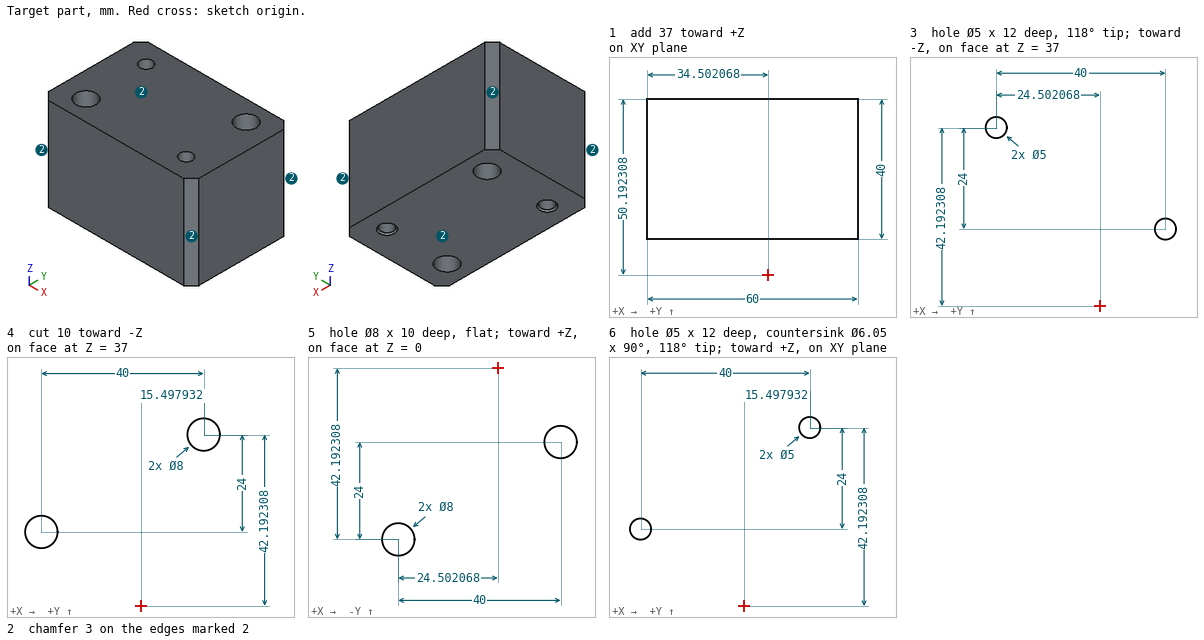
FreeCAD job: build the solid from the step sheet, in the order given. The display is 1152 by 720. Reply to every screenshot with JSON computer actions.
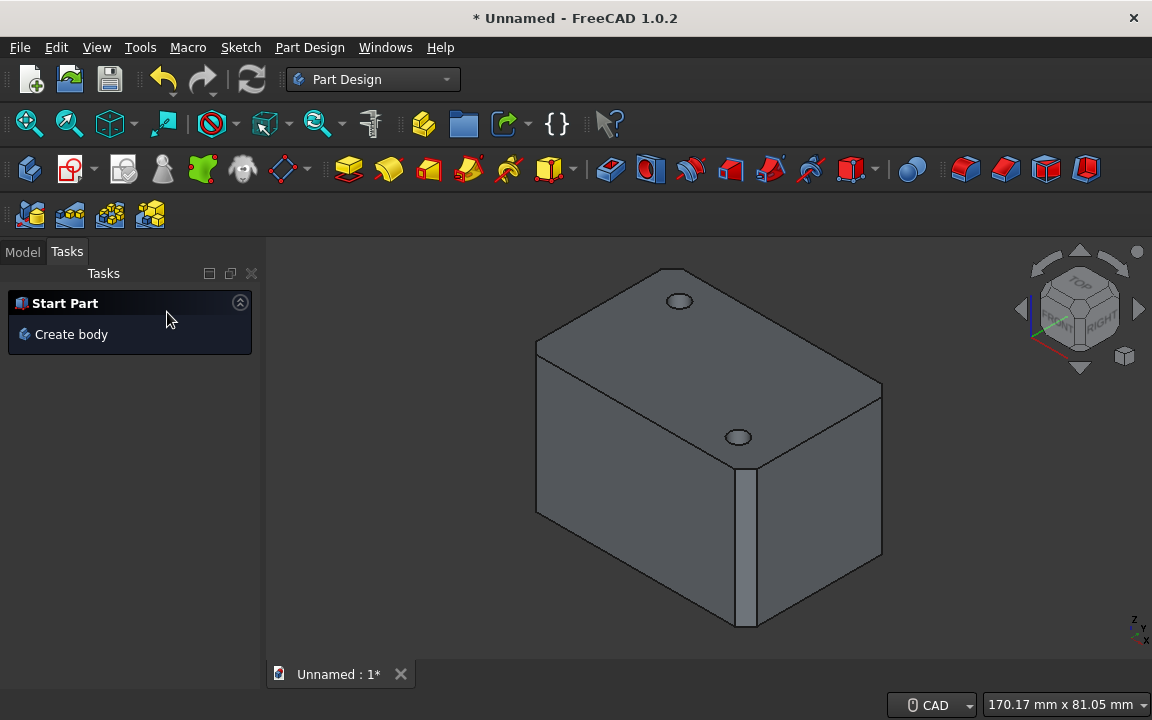
{"action": "left_click", "coordinate": [709, 368]}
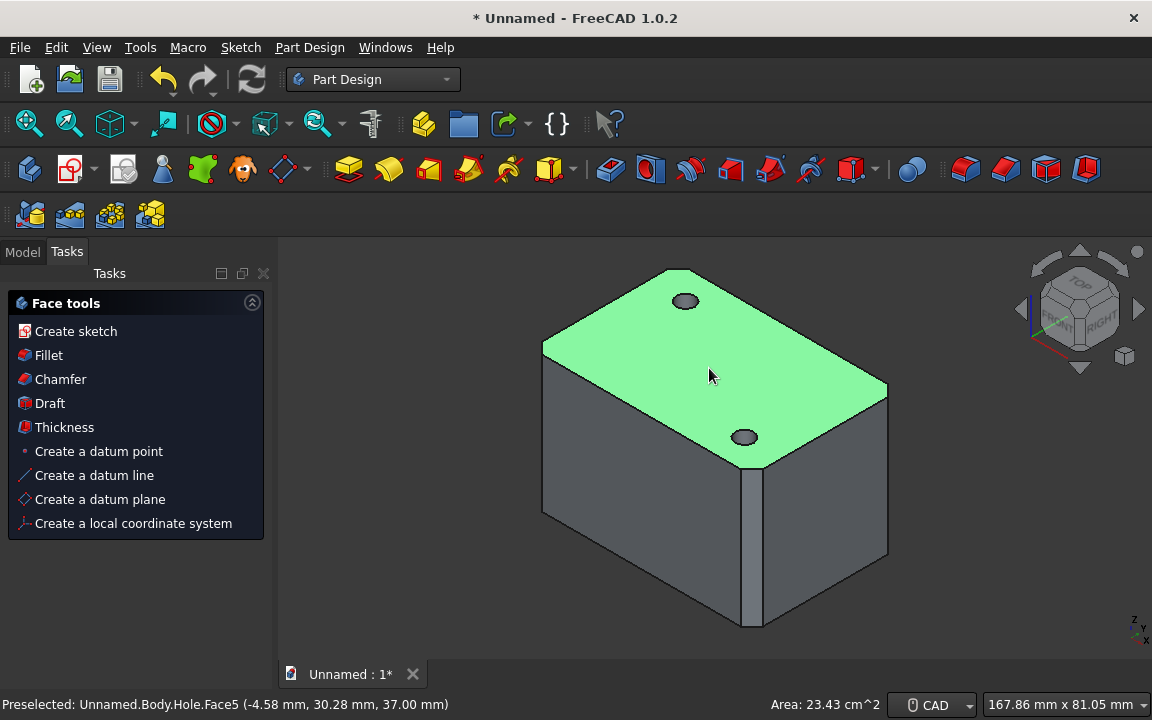
{"action": "left_click", "coordinate": [70, 170]}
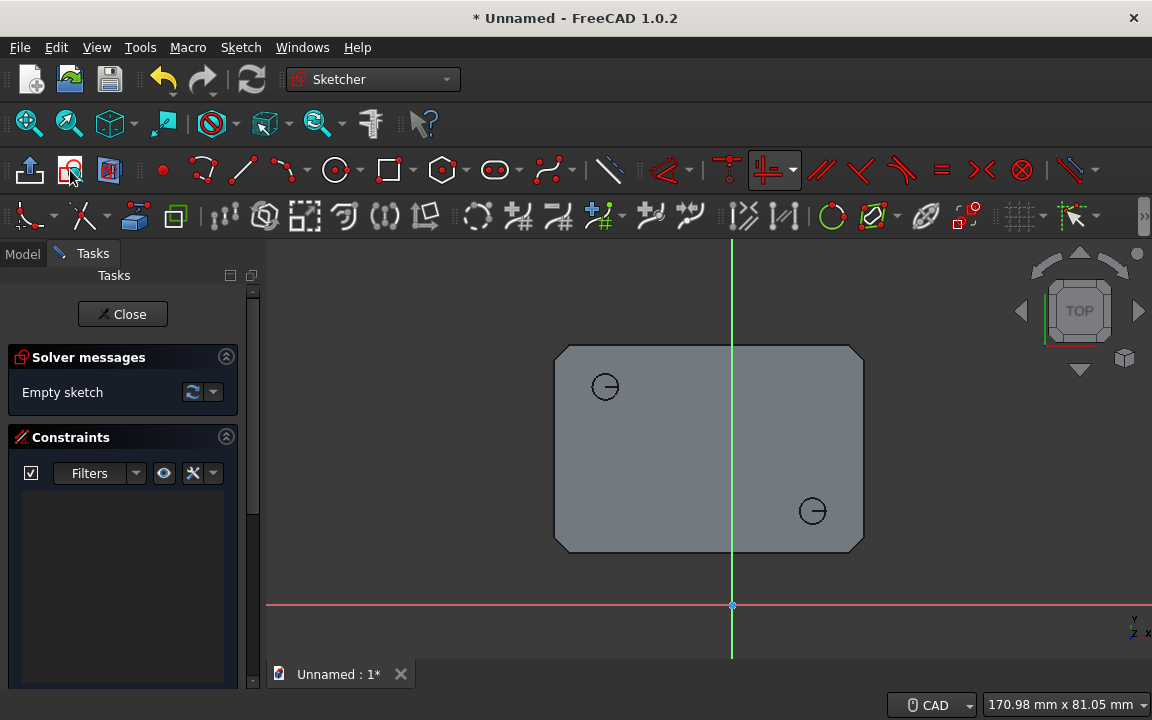
{"action": "left_click", "coordinate": [336, 170]}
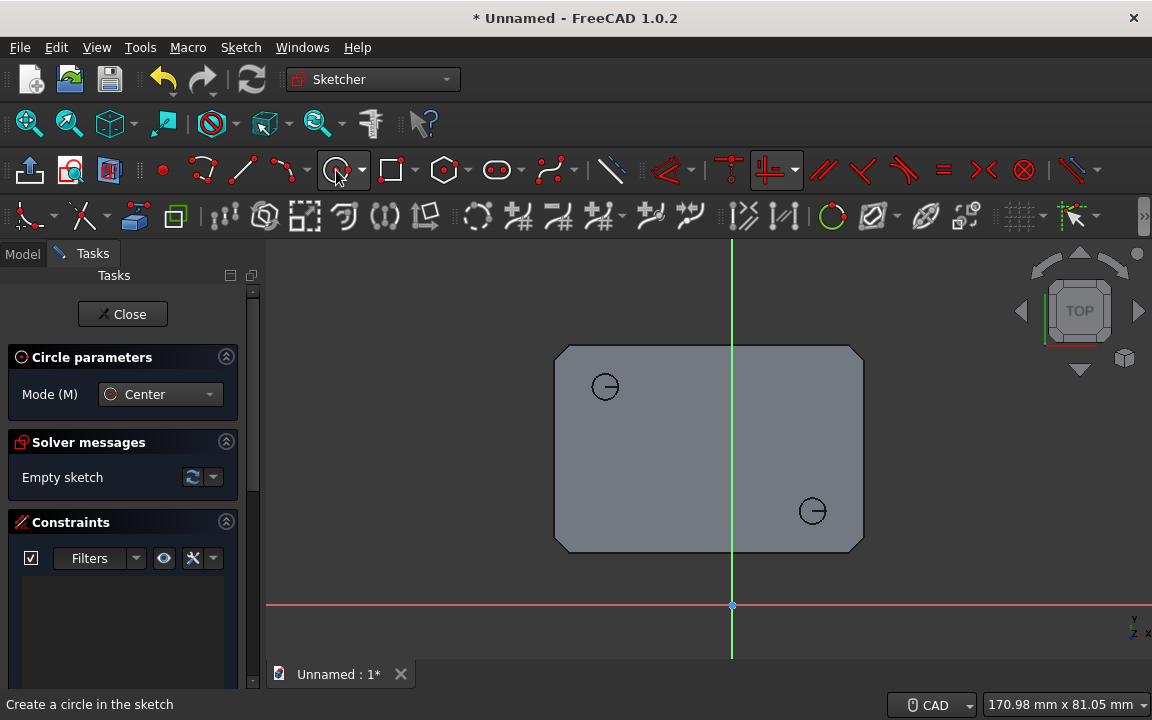
{"action": "left_click", "coordinate": [813, 387]}
{"action": "mouse_move", "coordinate": [827, 372]}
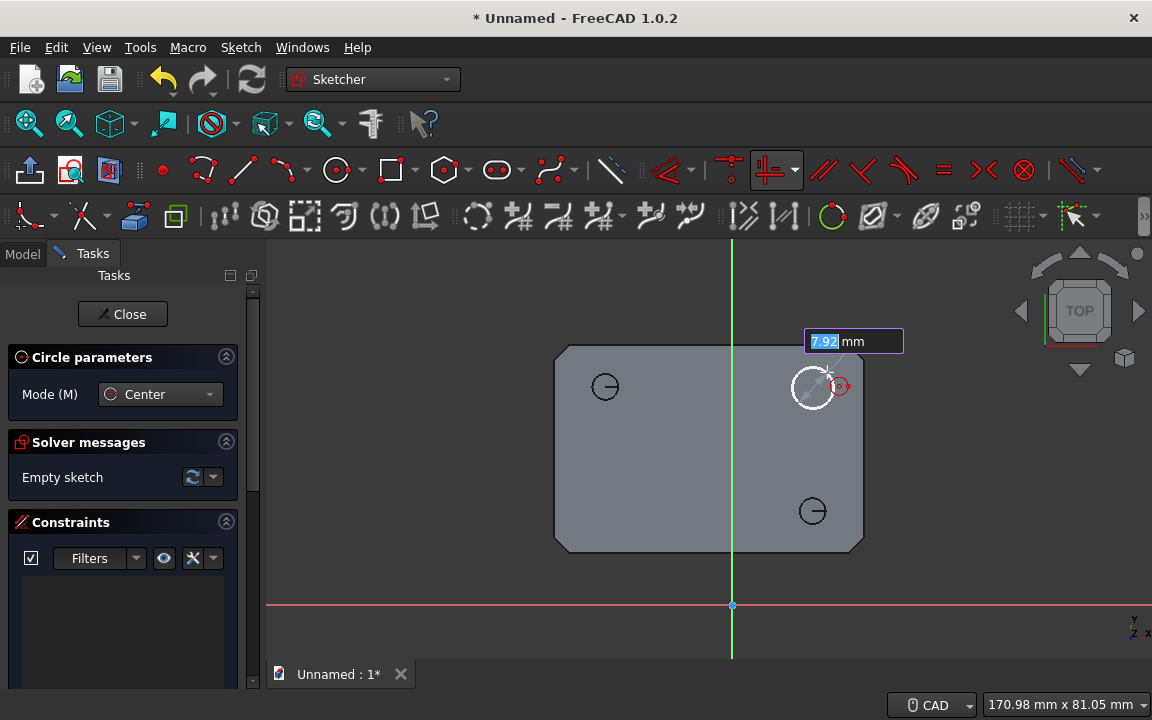
{"action": "type", "text": "8"}
{"action": "key", "text": "Return"}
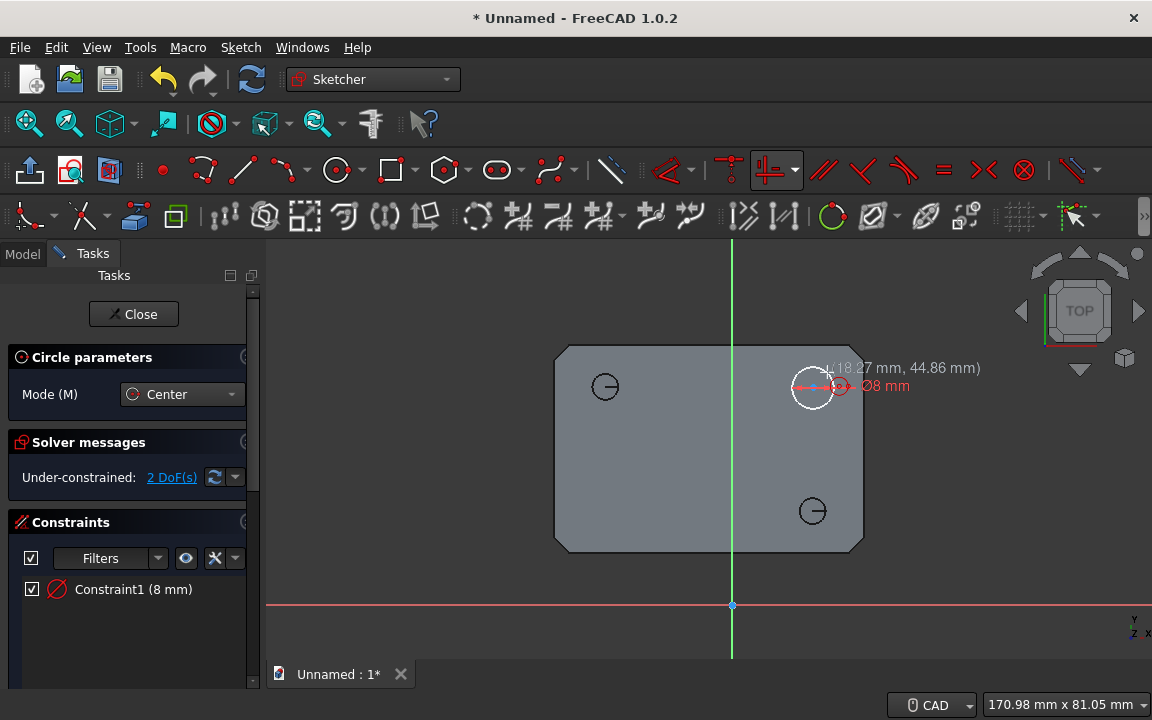
{"action": "left_click", "coordinate": [605, 511]}
{"action": "mouse_move", "coordinate": [620, 497]}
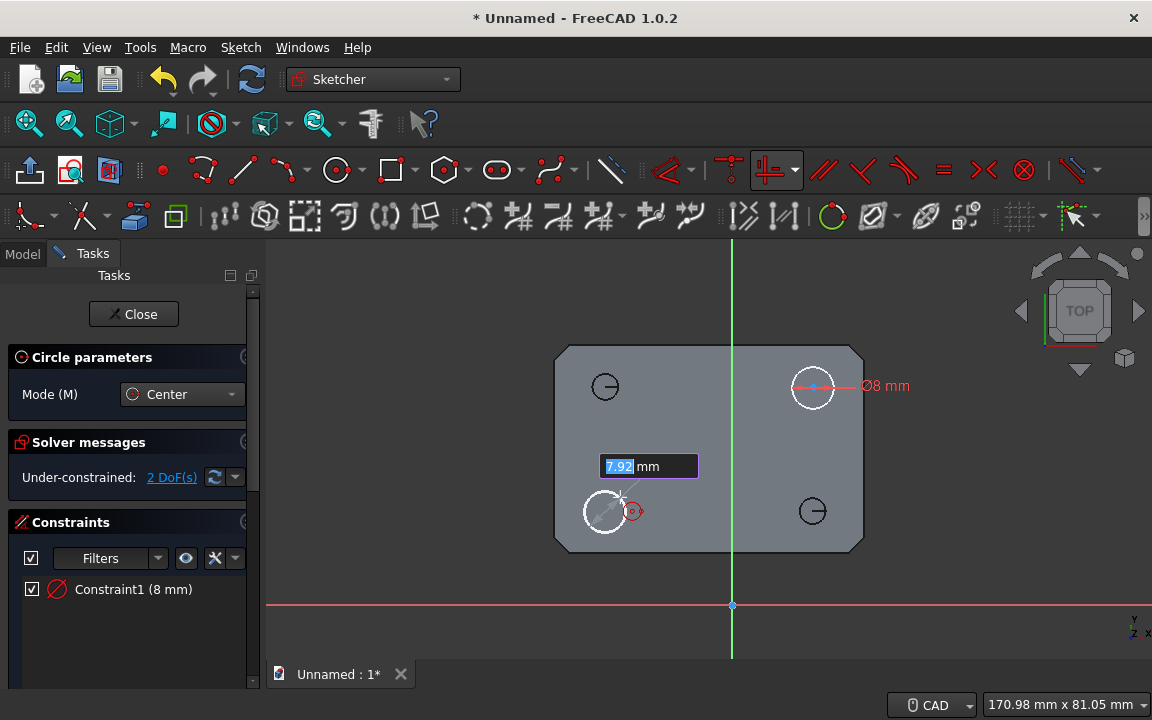
{"action": "type", "text": "8"}
{"action": "key", "text": "Return"}
{"action": "key", "text": "Escape"}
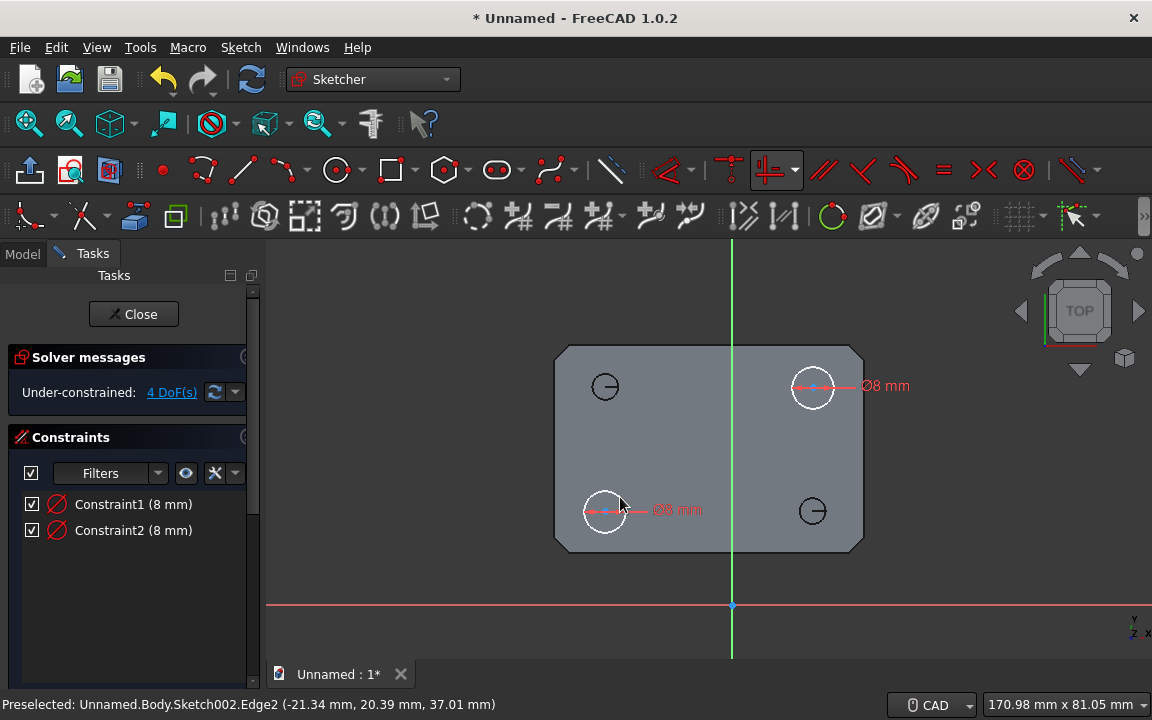
{"action": "left_click", "coordinate": [666, 170]}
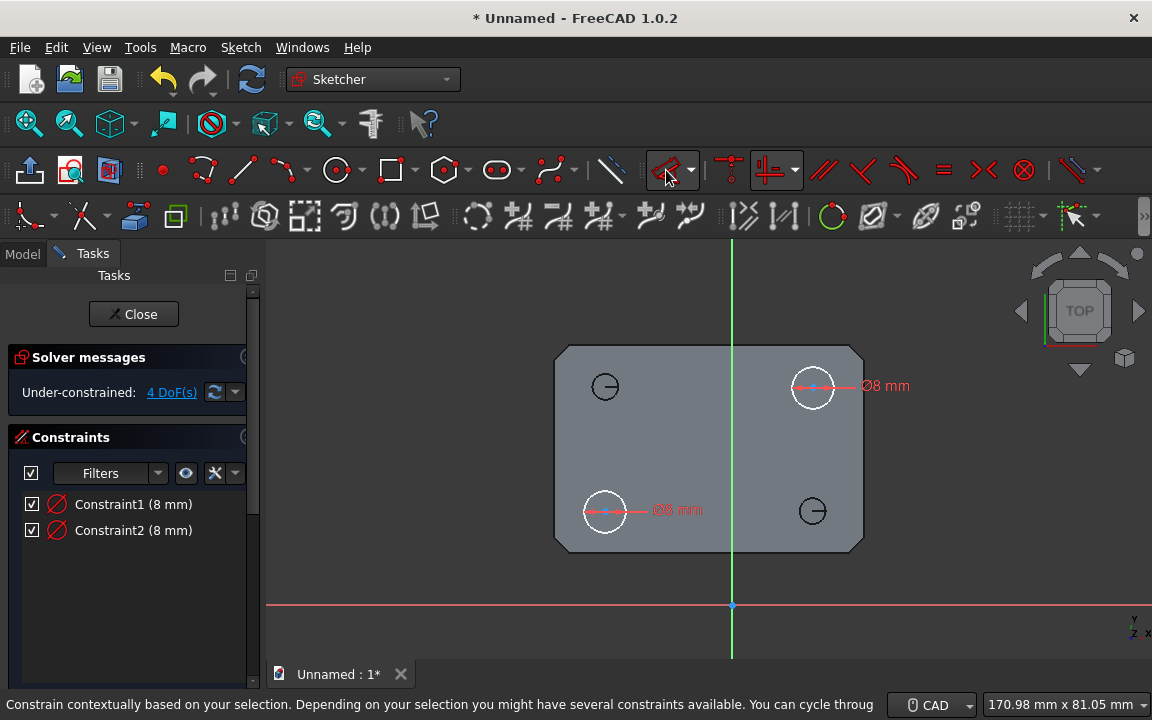
{"action": "left_click", "coordinate": [813, 388]}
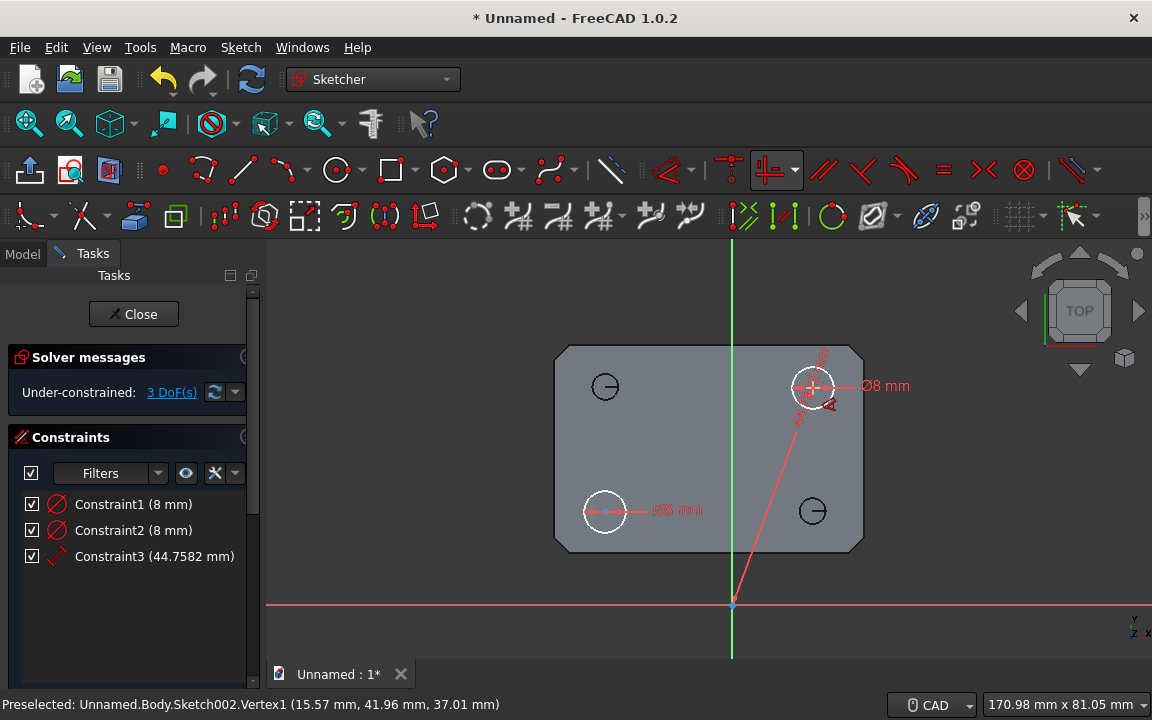
{"action": "left_click", "coordinate": [605, 512]}
{"action": "left_click", "coordinate": [709, 354]}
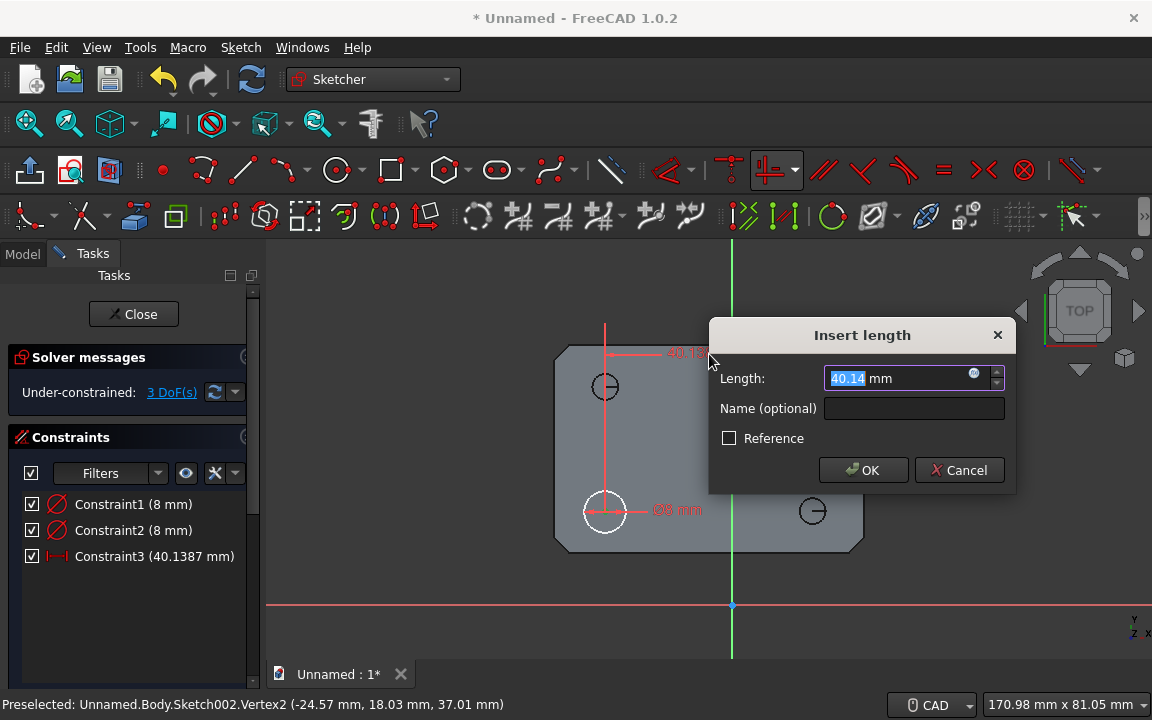
{"action": "type", "text": "40"}
{"action": "key", "text": "Return"}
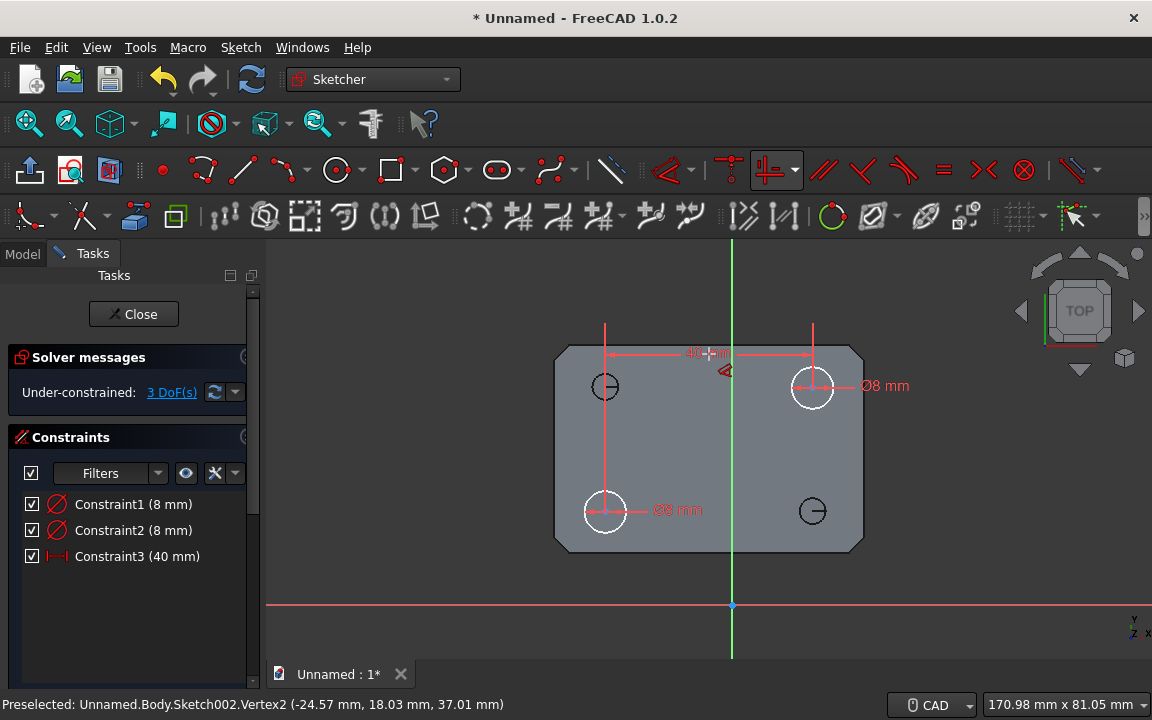
{"action": "left_click", "coordinate": [813, 388]}